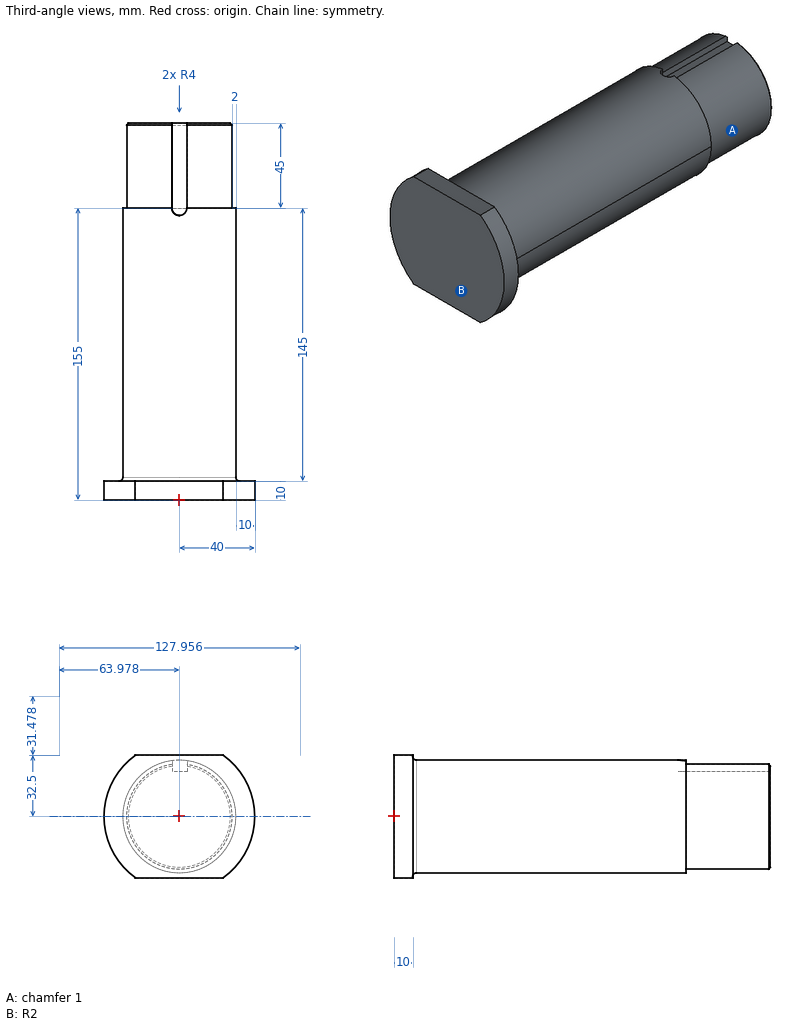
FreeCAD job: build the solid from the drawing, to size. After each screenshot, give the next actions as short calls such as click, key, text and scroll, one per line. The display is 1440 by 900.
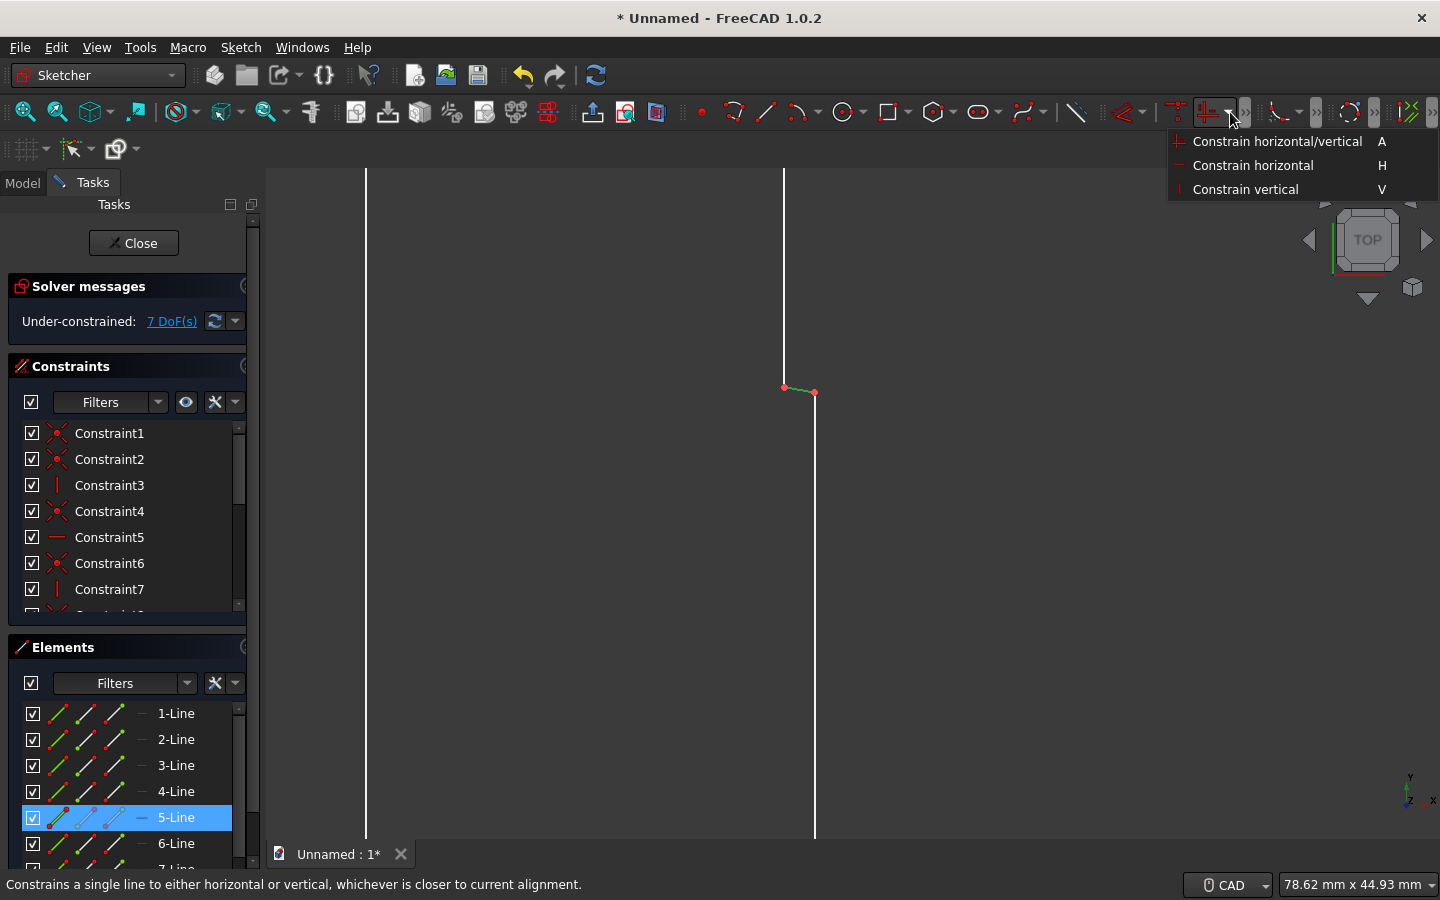
click(1303, 165)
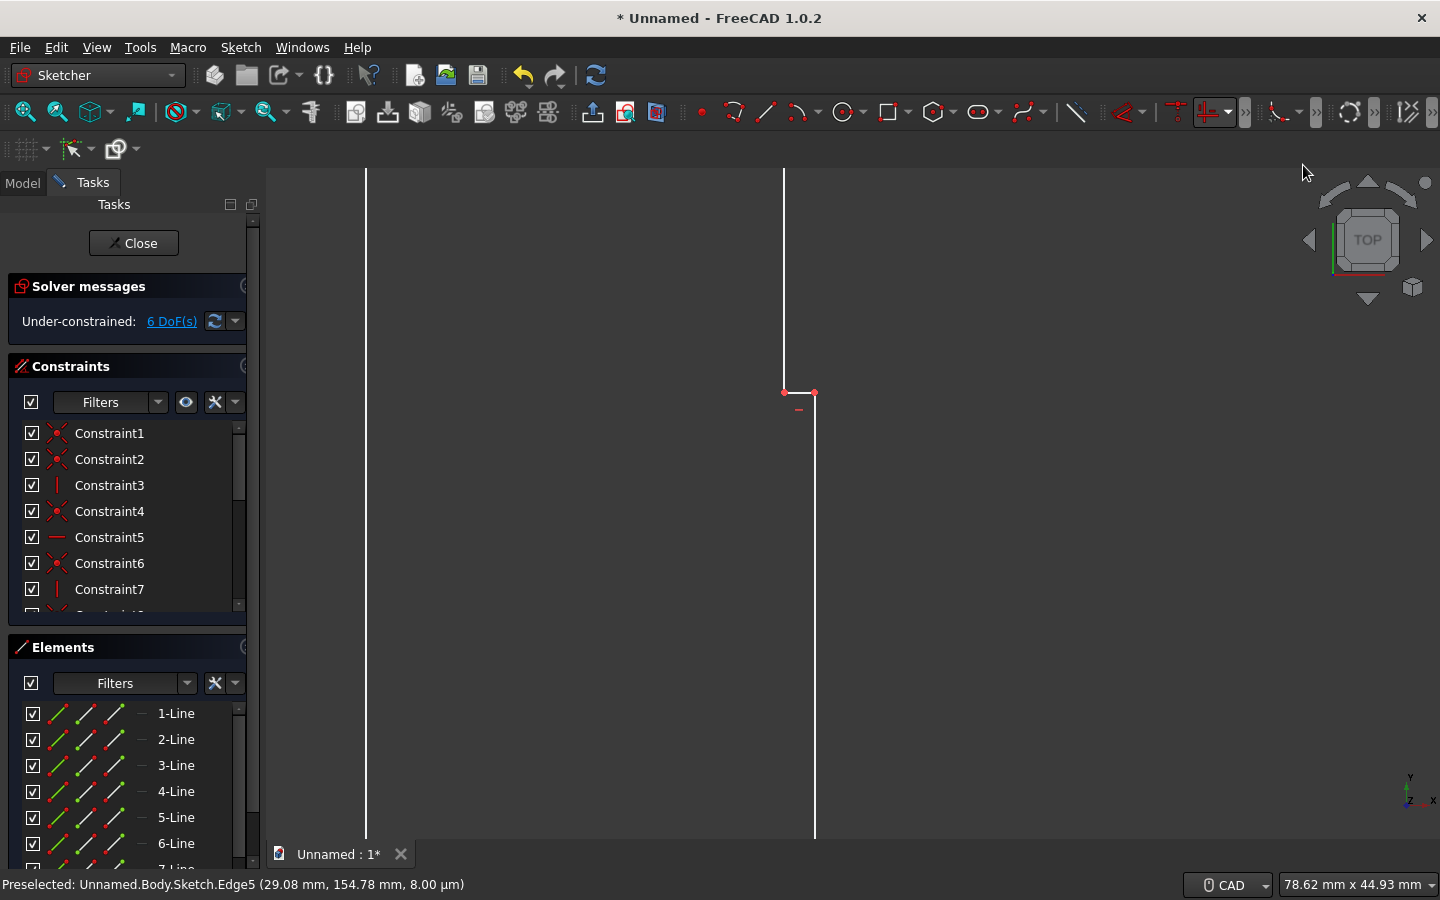
click(1122, 112)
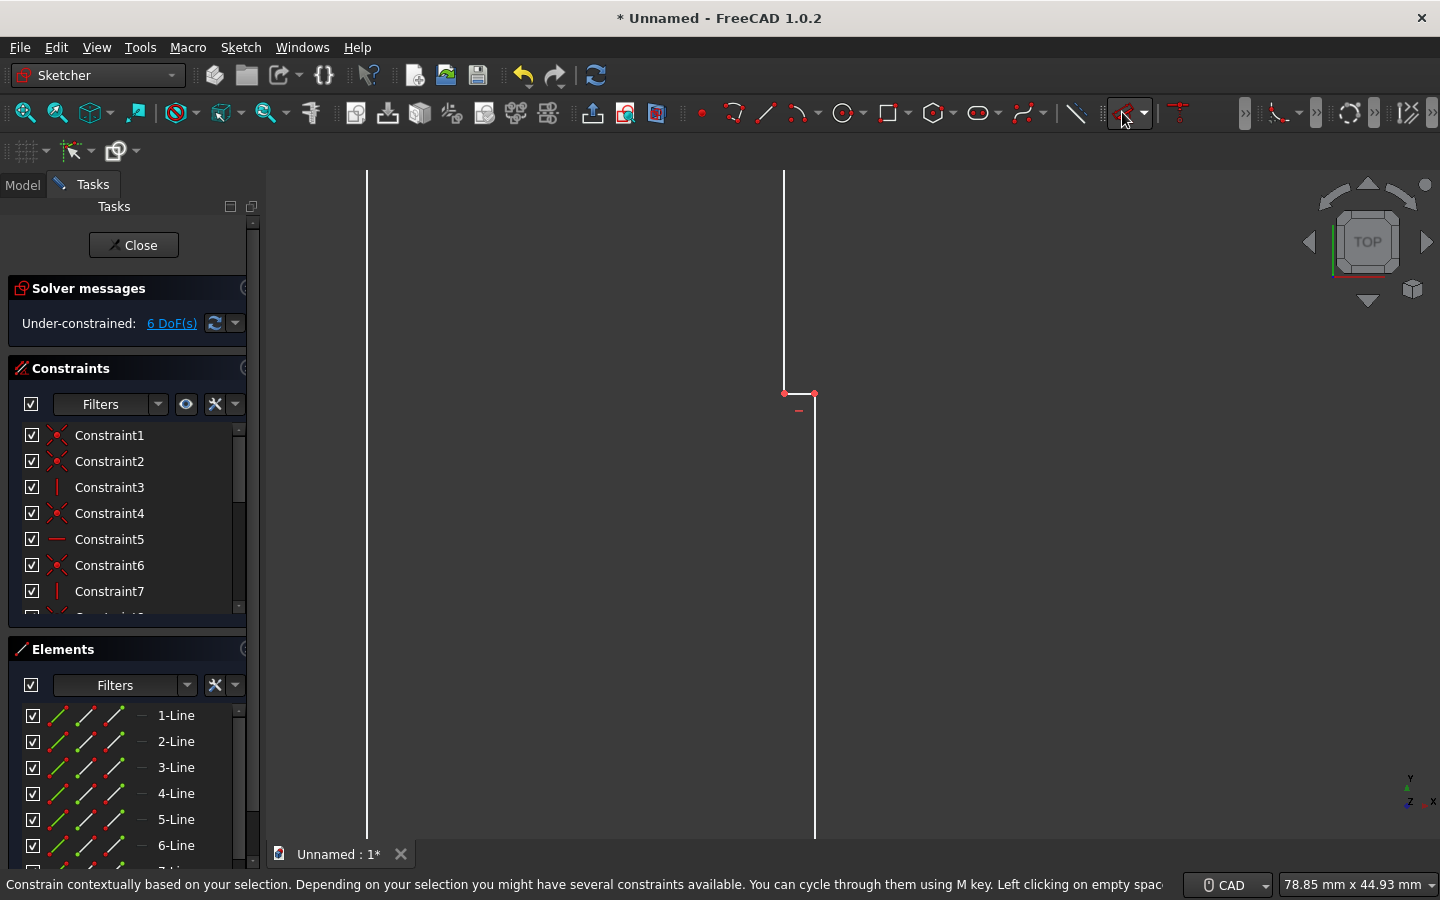
scroll(806, 394, up, 3)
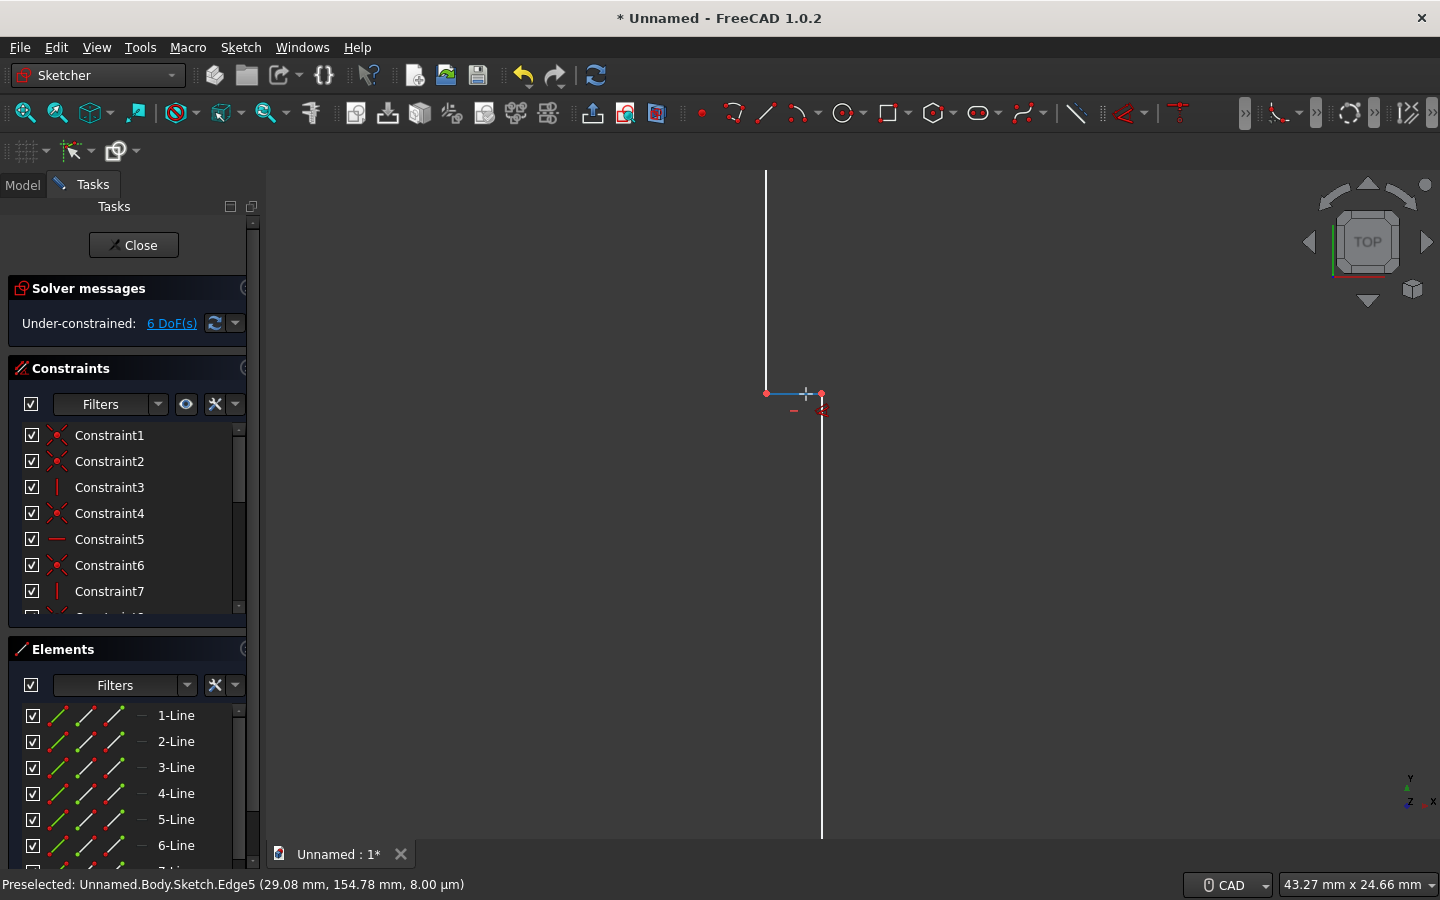
click(805, 394)
click(794, 360)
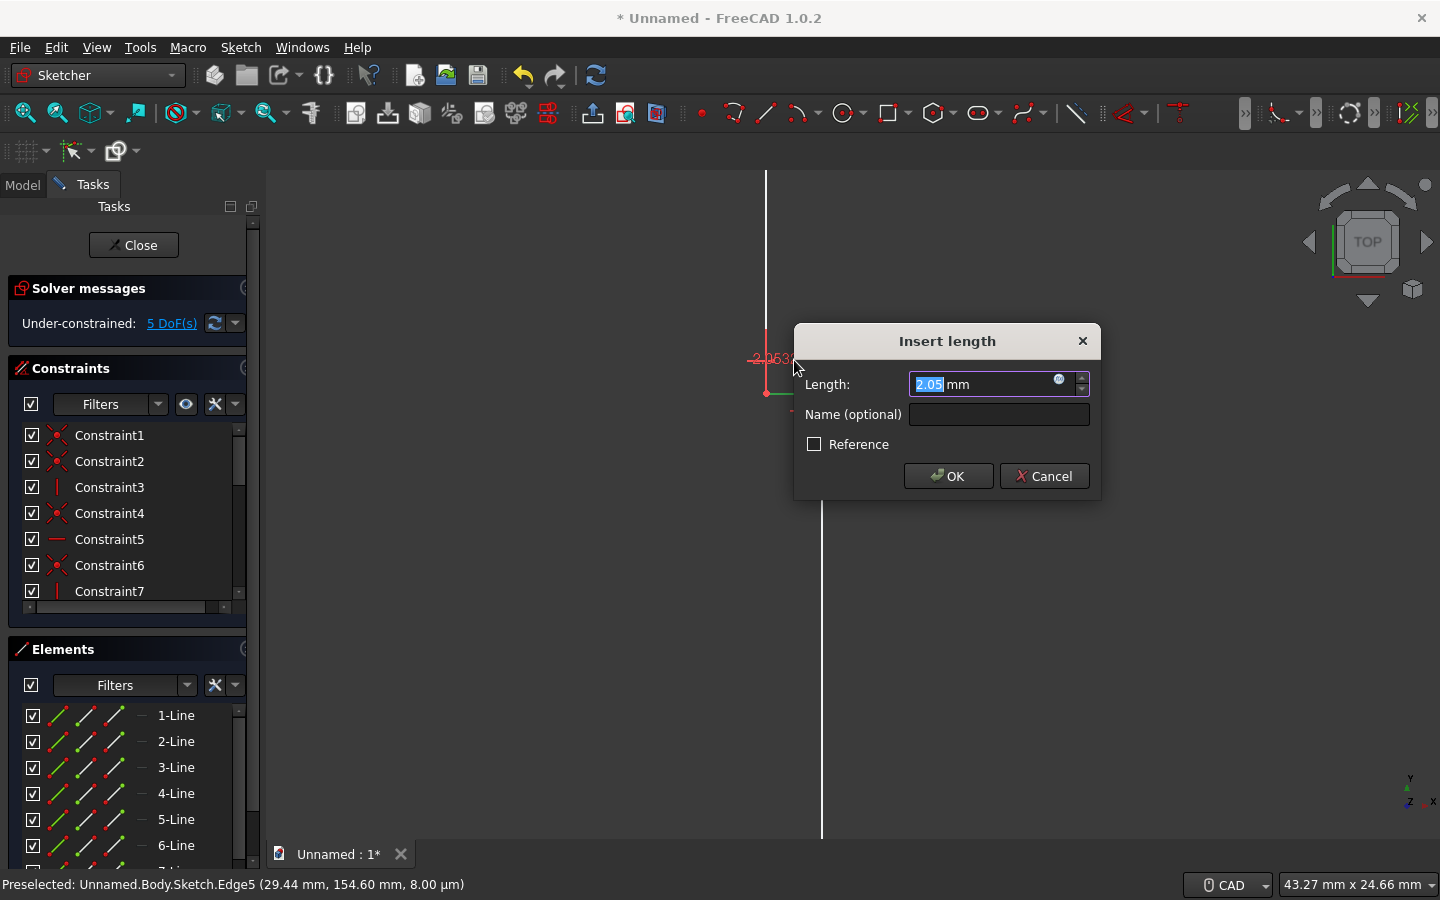
text(2)
key(Return)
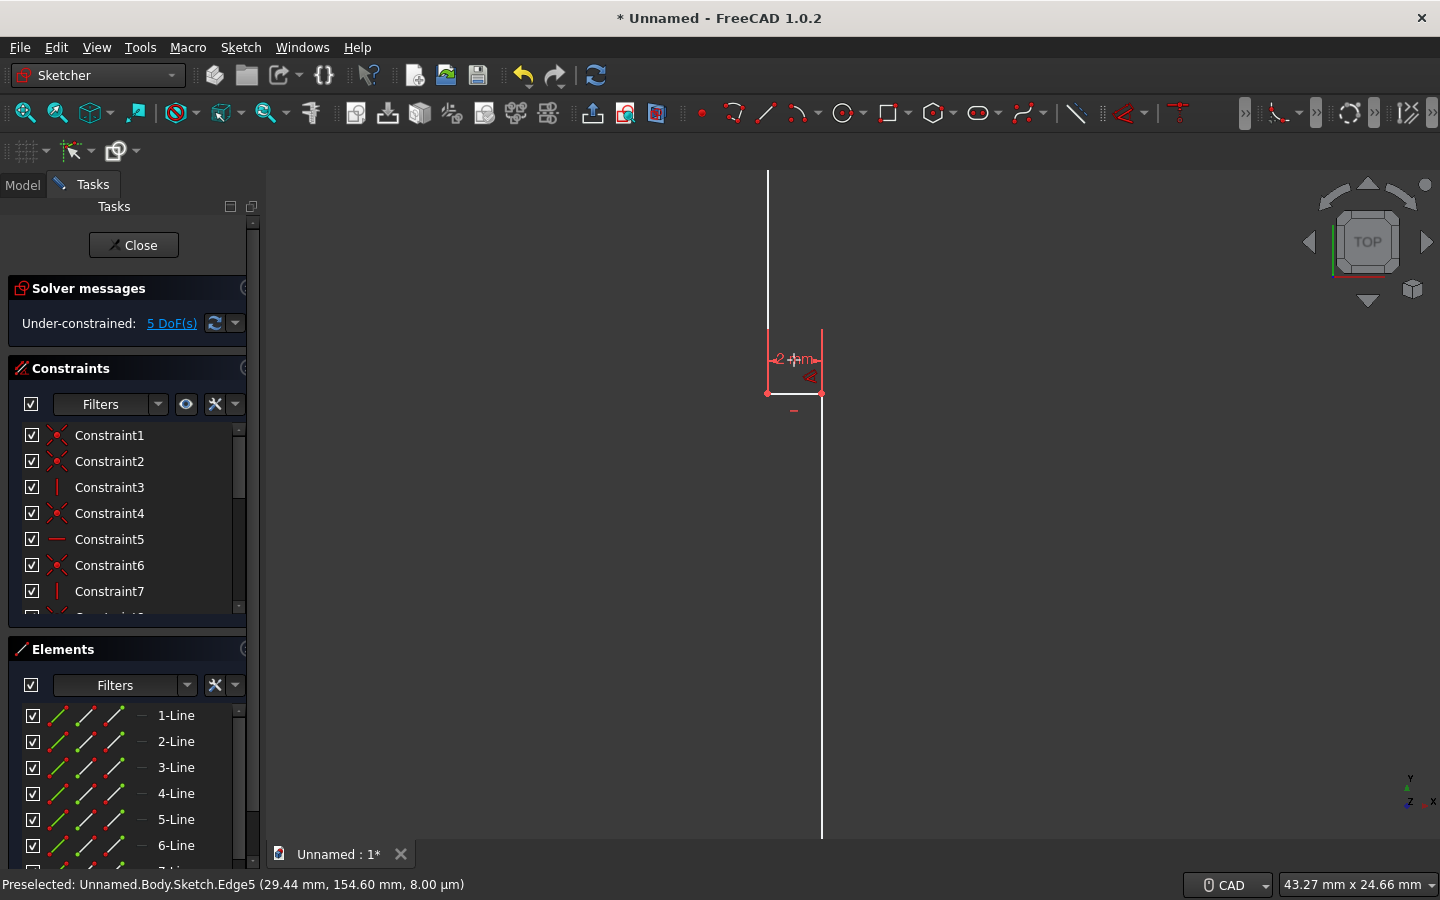
scroll(803, 395, down, 13)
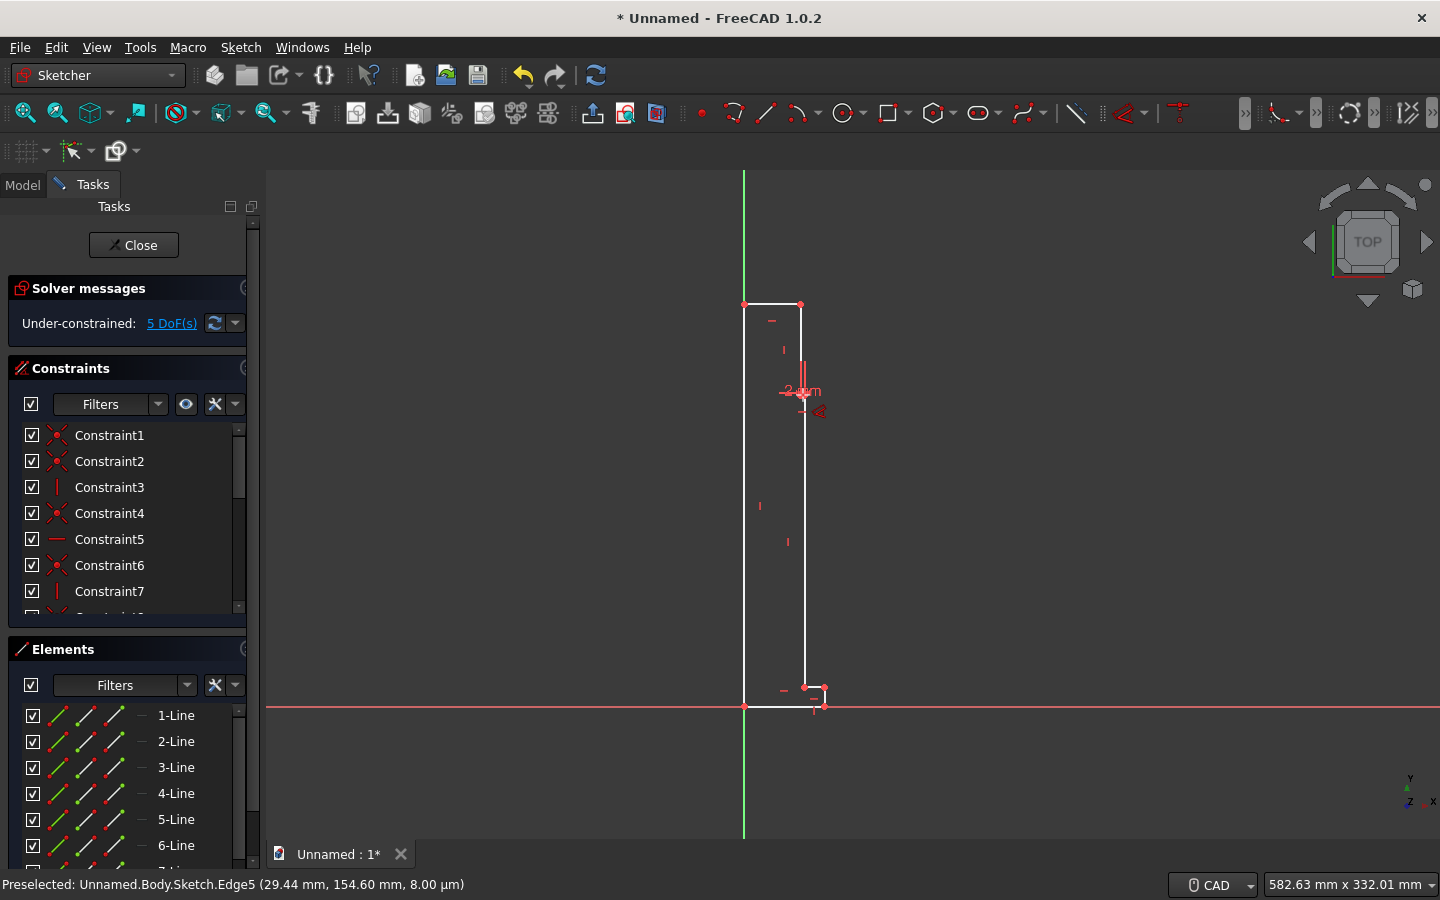
click(768, 707)
click(785, 741)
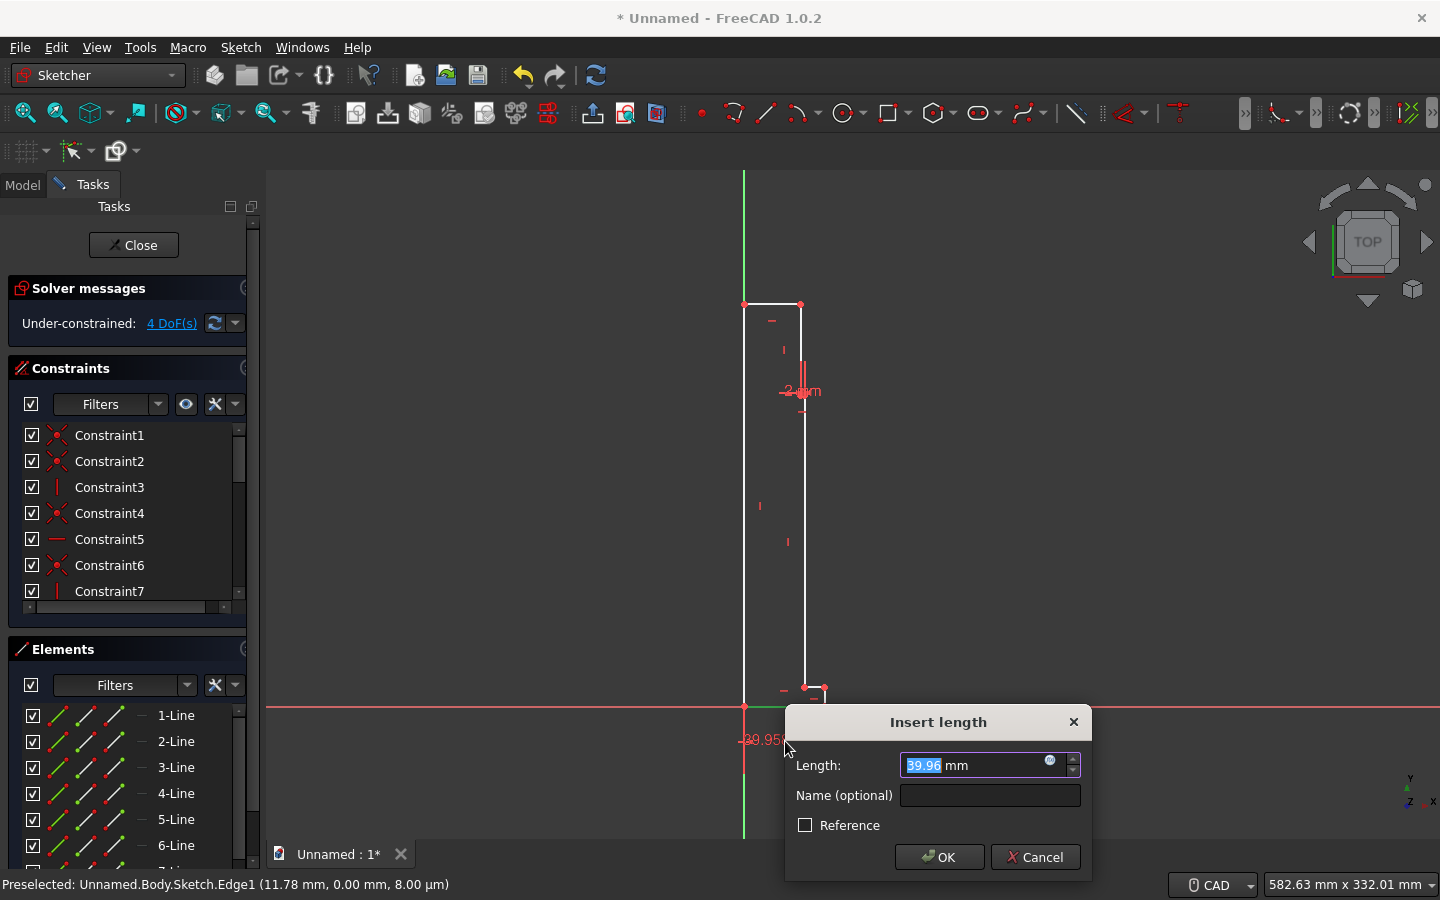
text(40)
key(Return)